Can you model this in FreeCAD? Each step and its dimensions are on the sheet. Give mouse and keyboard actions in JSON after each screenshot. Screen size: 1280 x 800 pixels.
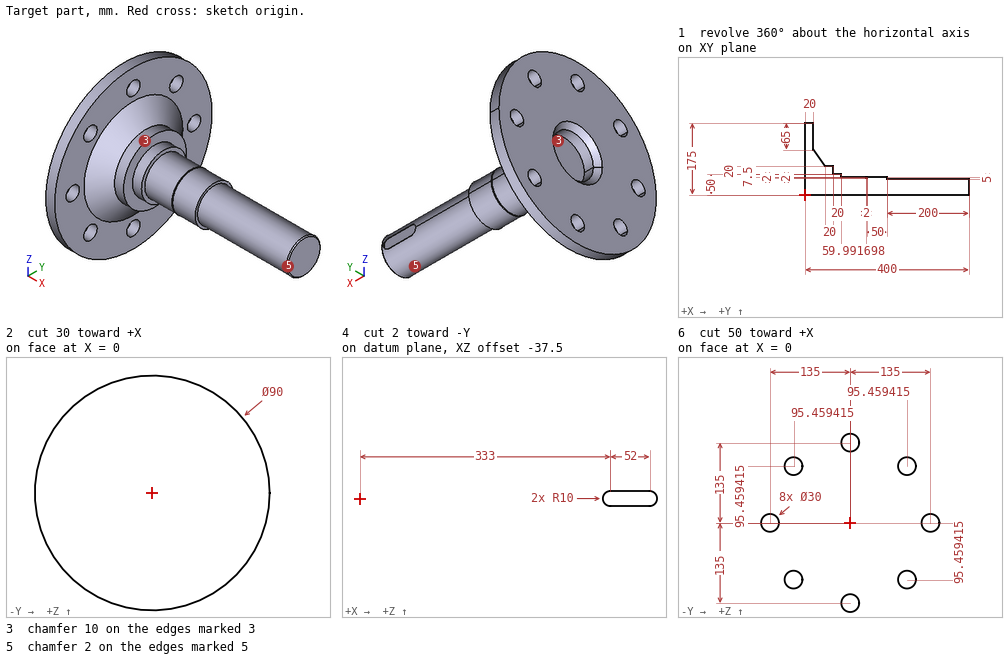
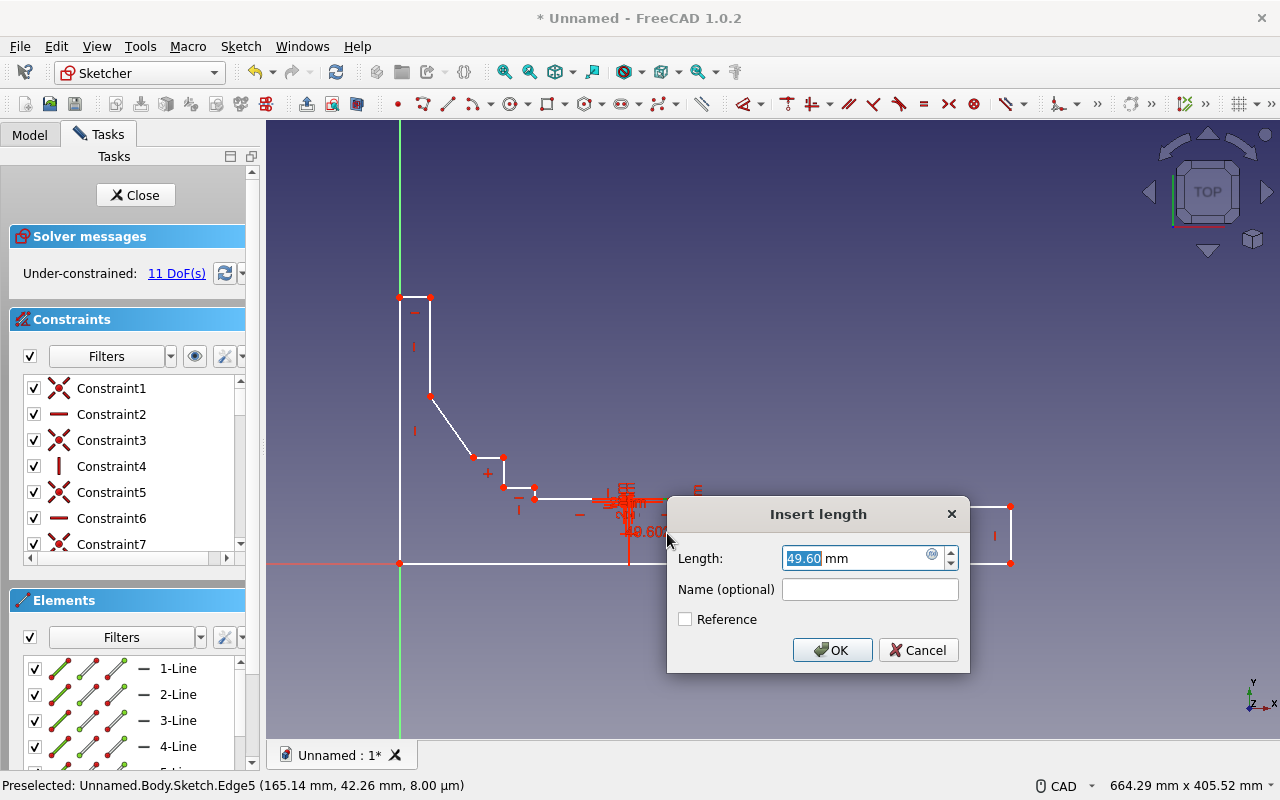
{"action": "type", "text": "50"}
{"action": "key", "text": "Return"}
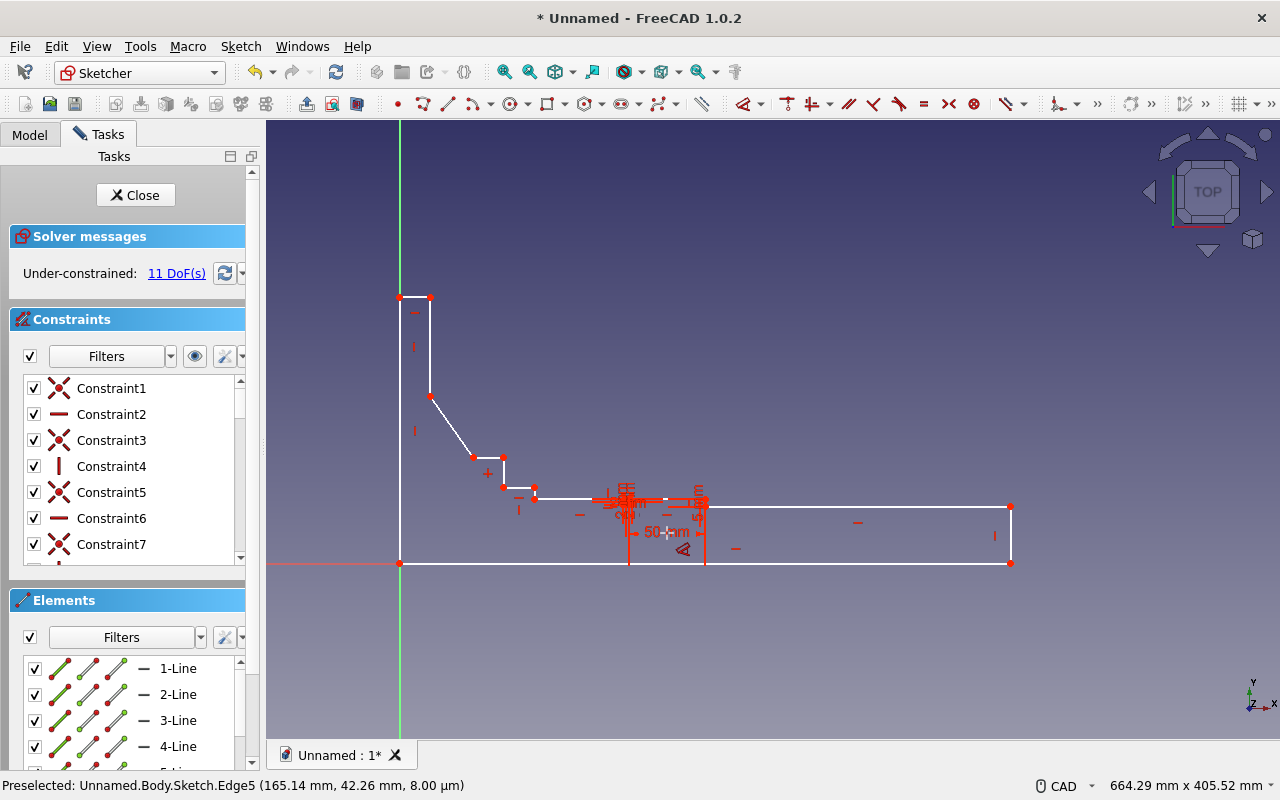
{"action": "scroll", "coordinate": [526, 488], "scroll_direction": "up", "scroll_amount": 3}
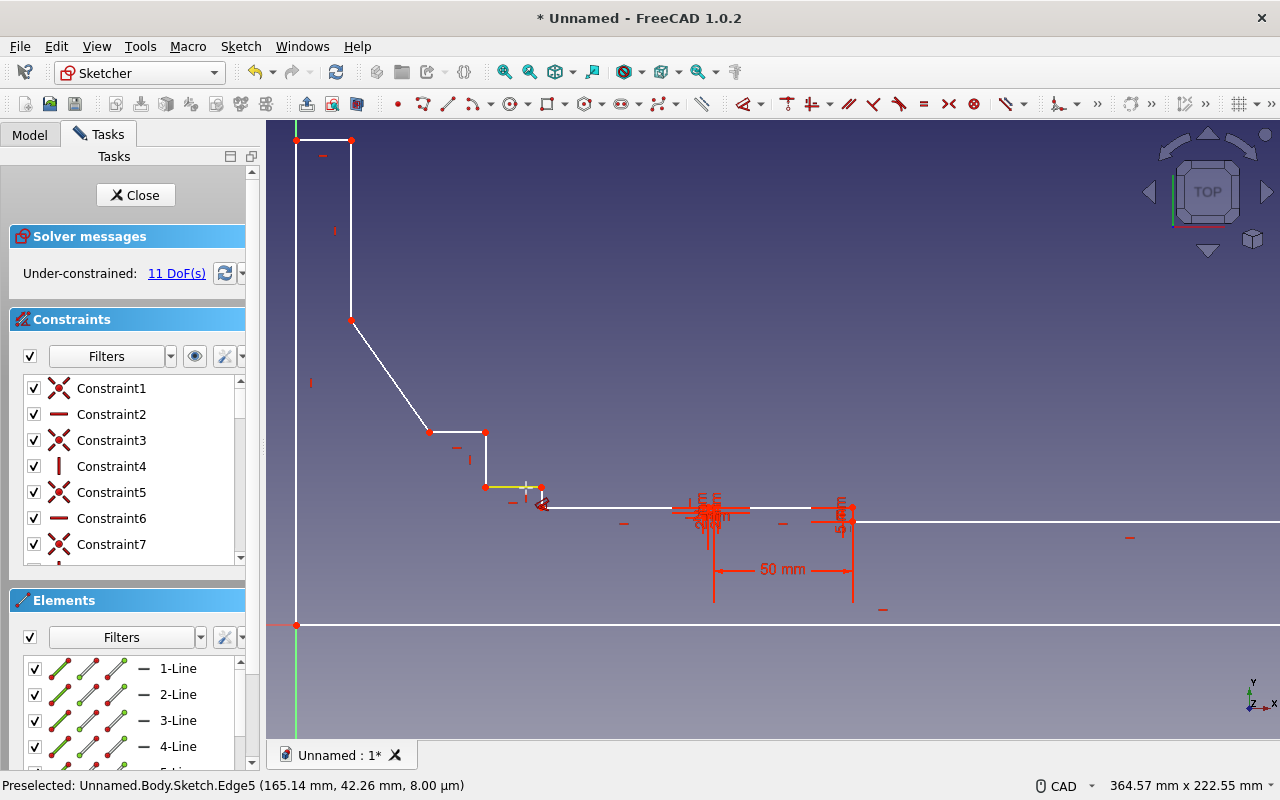
{"action": "left_click", "coordinate": [525, 487]}
{"action": "left_click", "coordinate": [514, 521]}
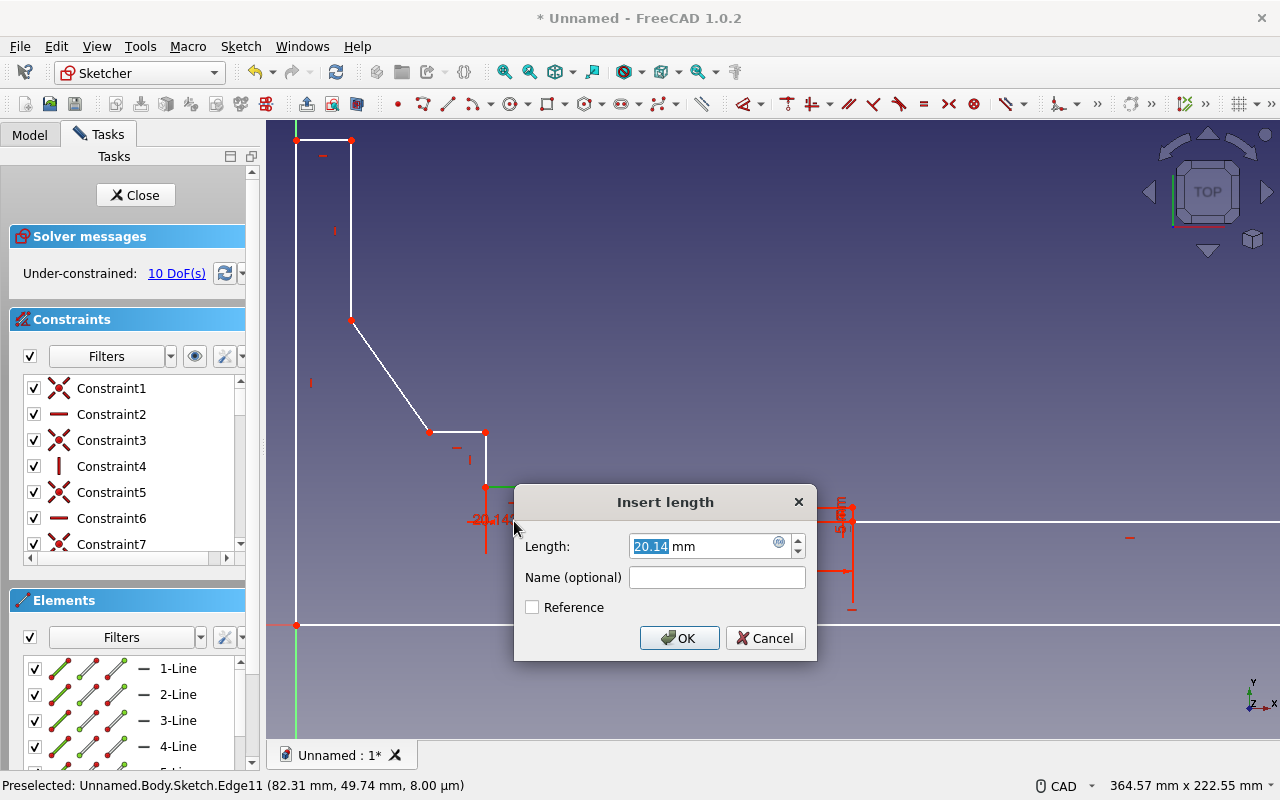
{"action": "type", "text": "20"}
{"action": "key", "text": "Return"}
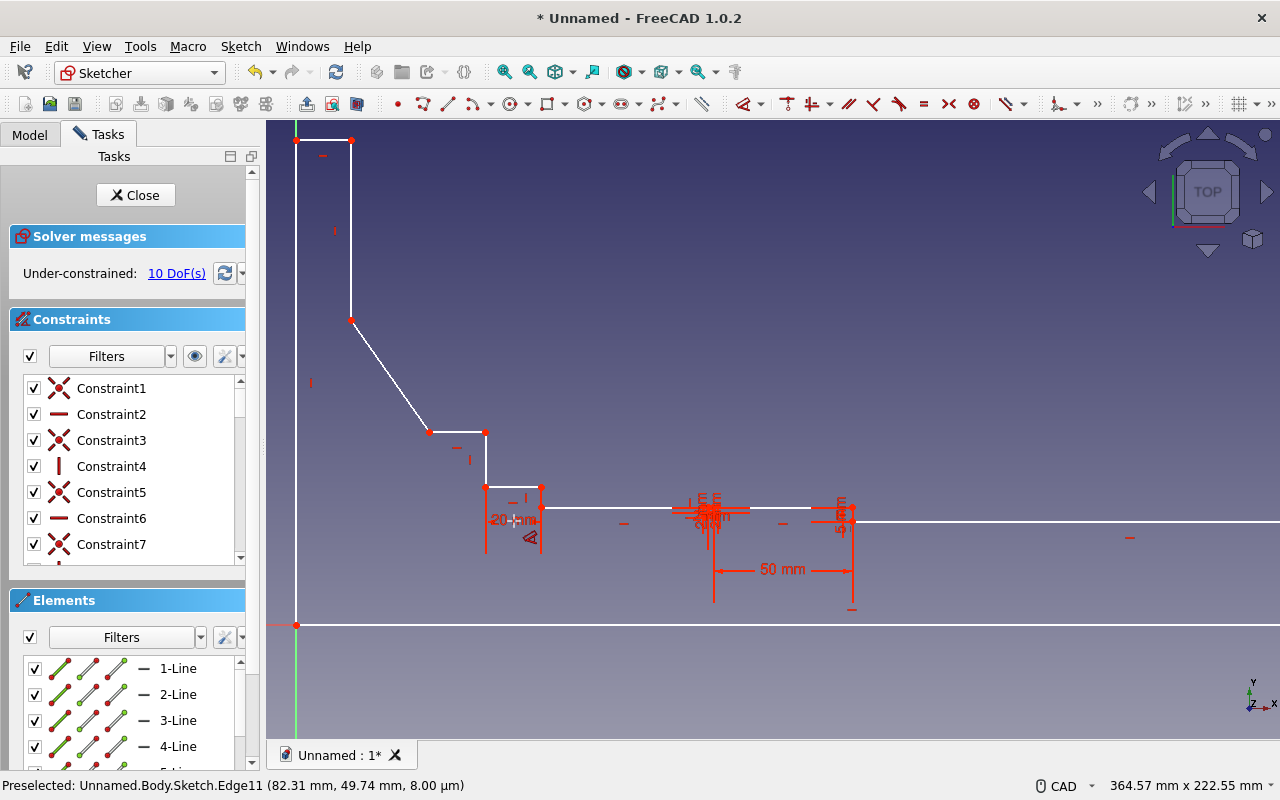
{"action": "left_click", "coordinate": [486, 471]}
{"action": "left_click", "coordinate": [452, 460]}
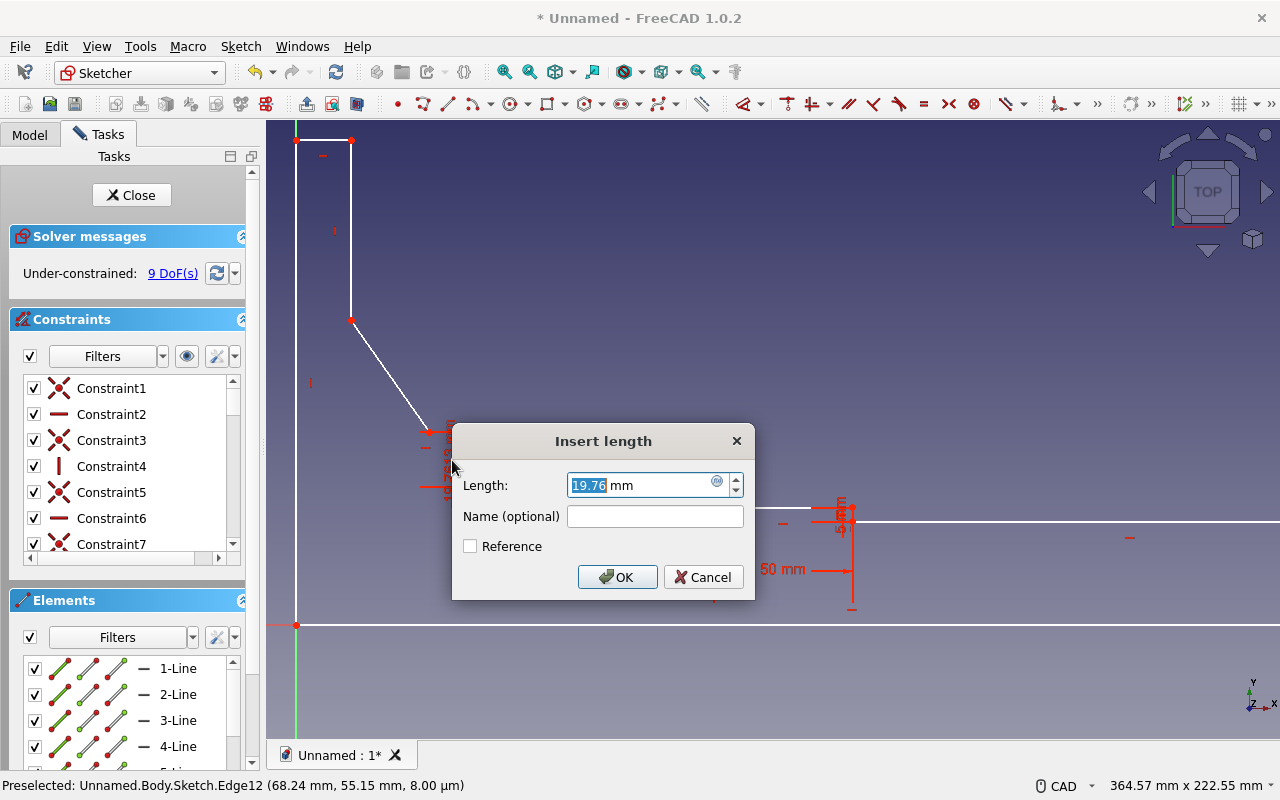
{"action": "type", "text": "20"}
{"action": "key", "text": "Return"}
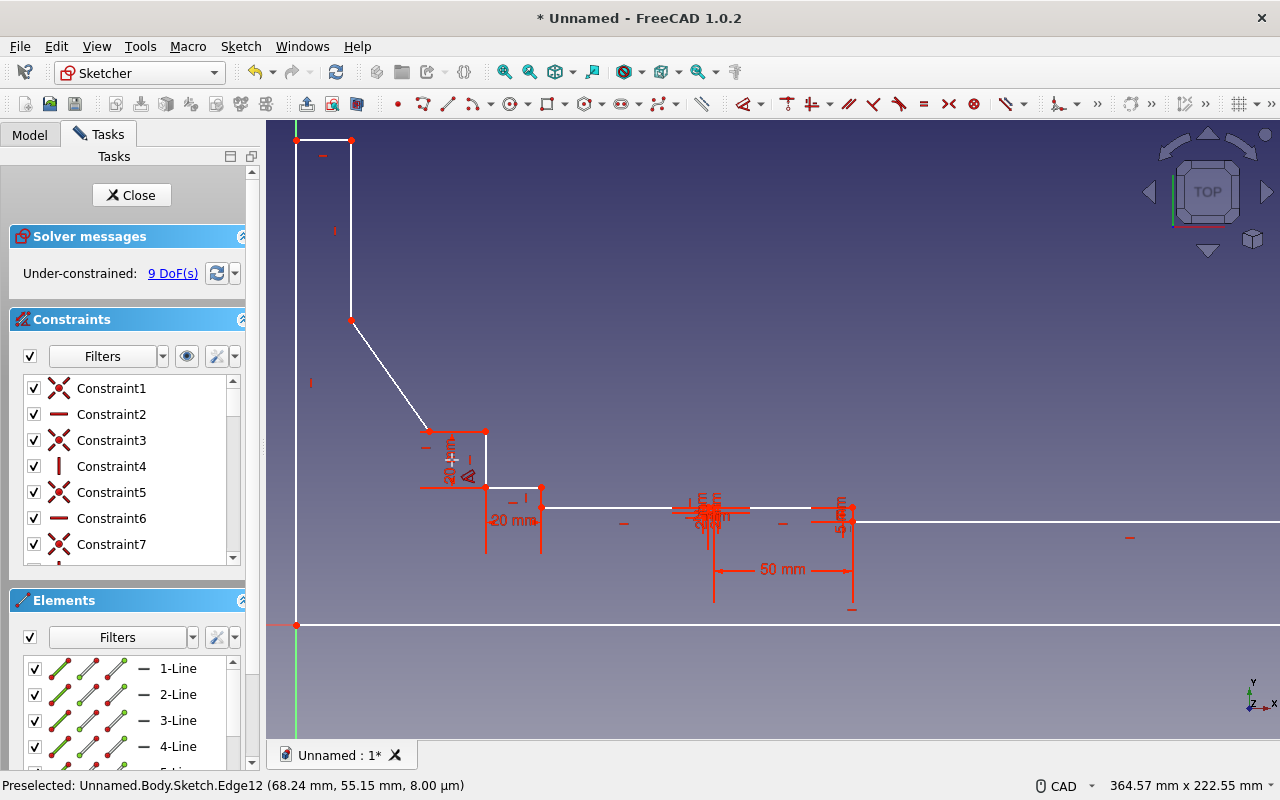
{"action": "left_click", "coordinate": [469, 432]}
{"action": "left_click", "coordinate": [458, 398]}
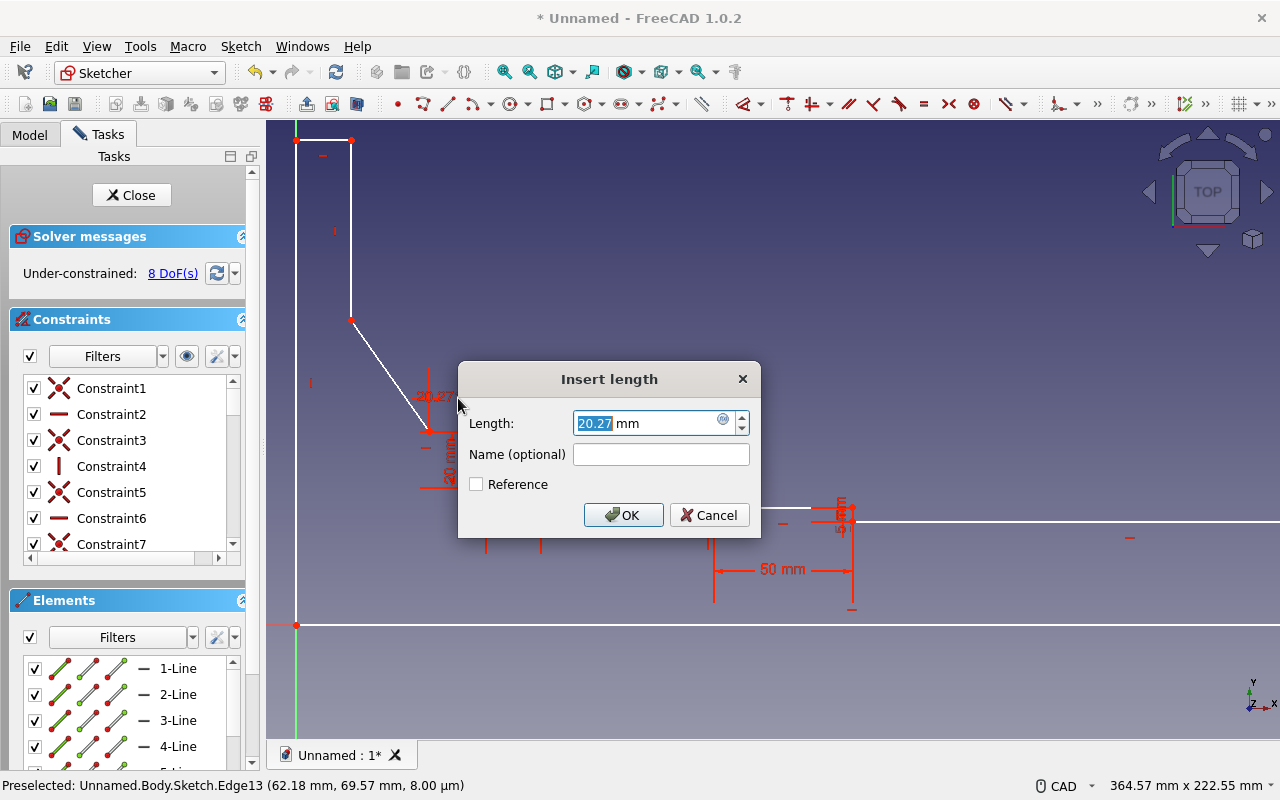
{"action": "type", "text": "20"}
{"action": "key", "text": "Return"}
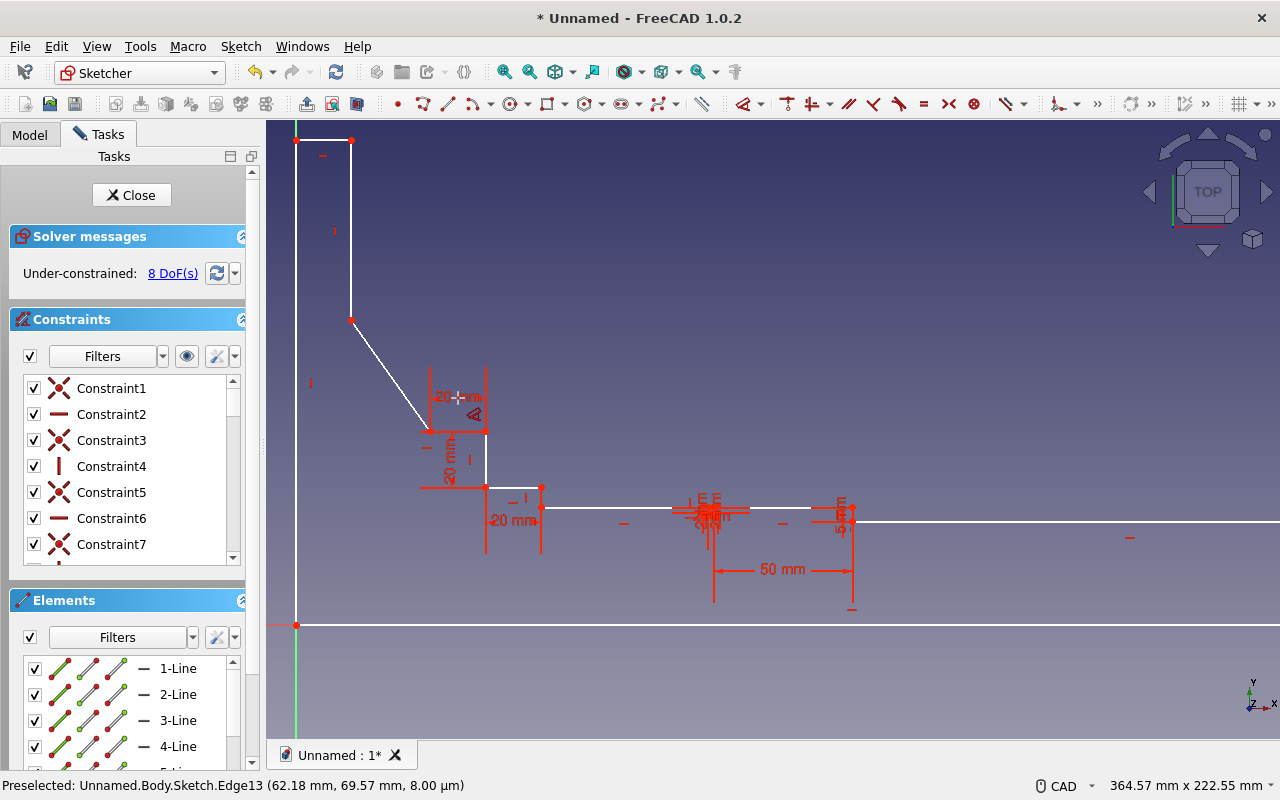
{"action": "left_click", "coordinate": [351, 267]}
{"action": "left_click", "coordinate": [317, 234]}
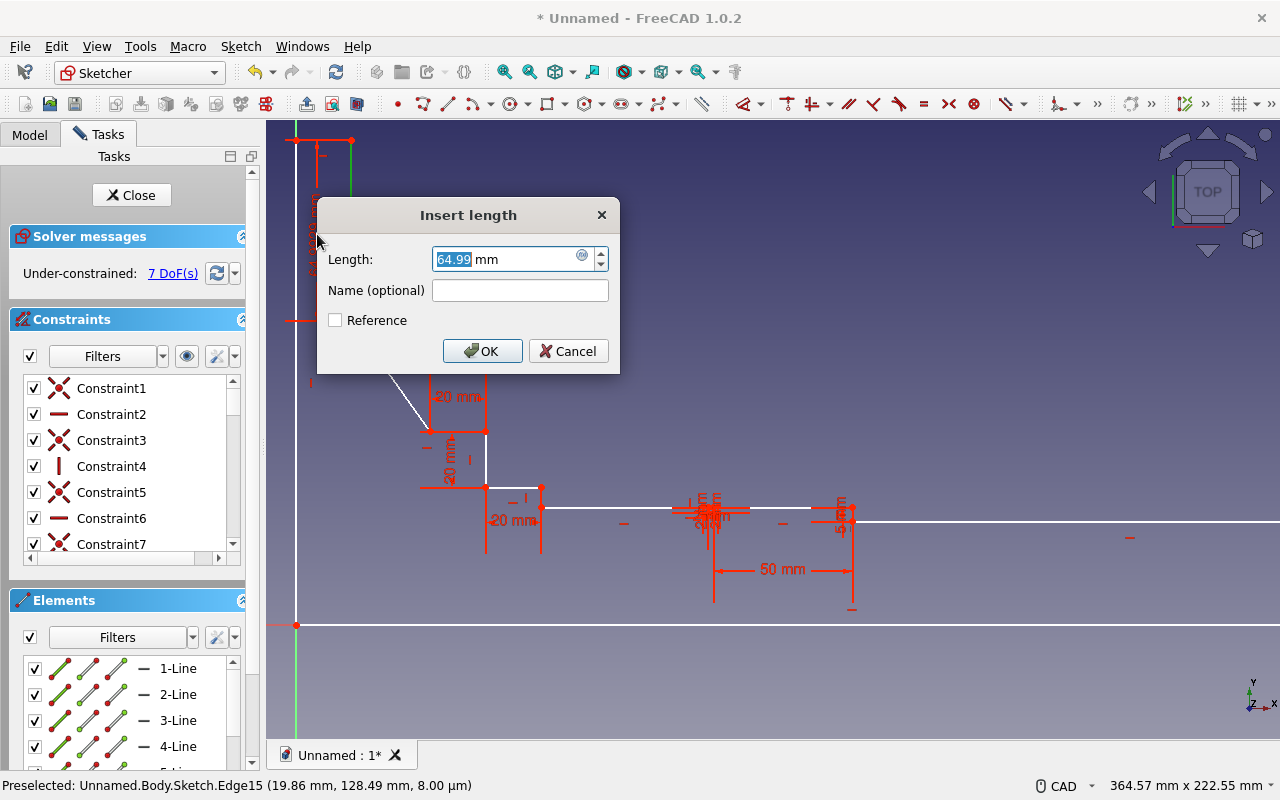
{"action": "type", "text": "65"}
{"action": "key", "text": "Return"}